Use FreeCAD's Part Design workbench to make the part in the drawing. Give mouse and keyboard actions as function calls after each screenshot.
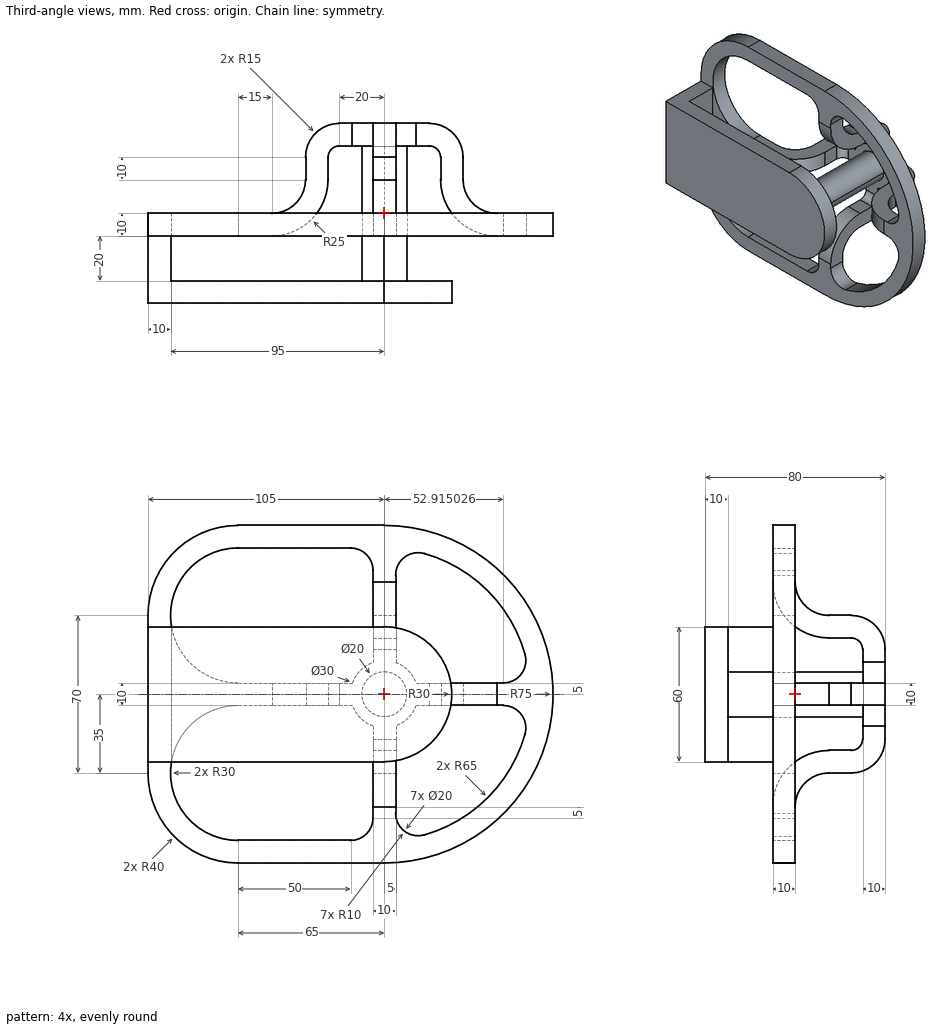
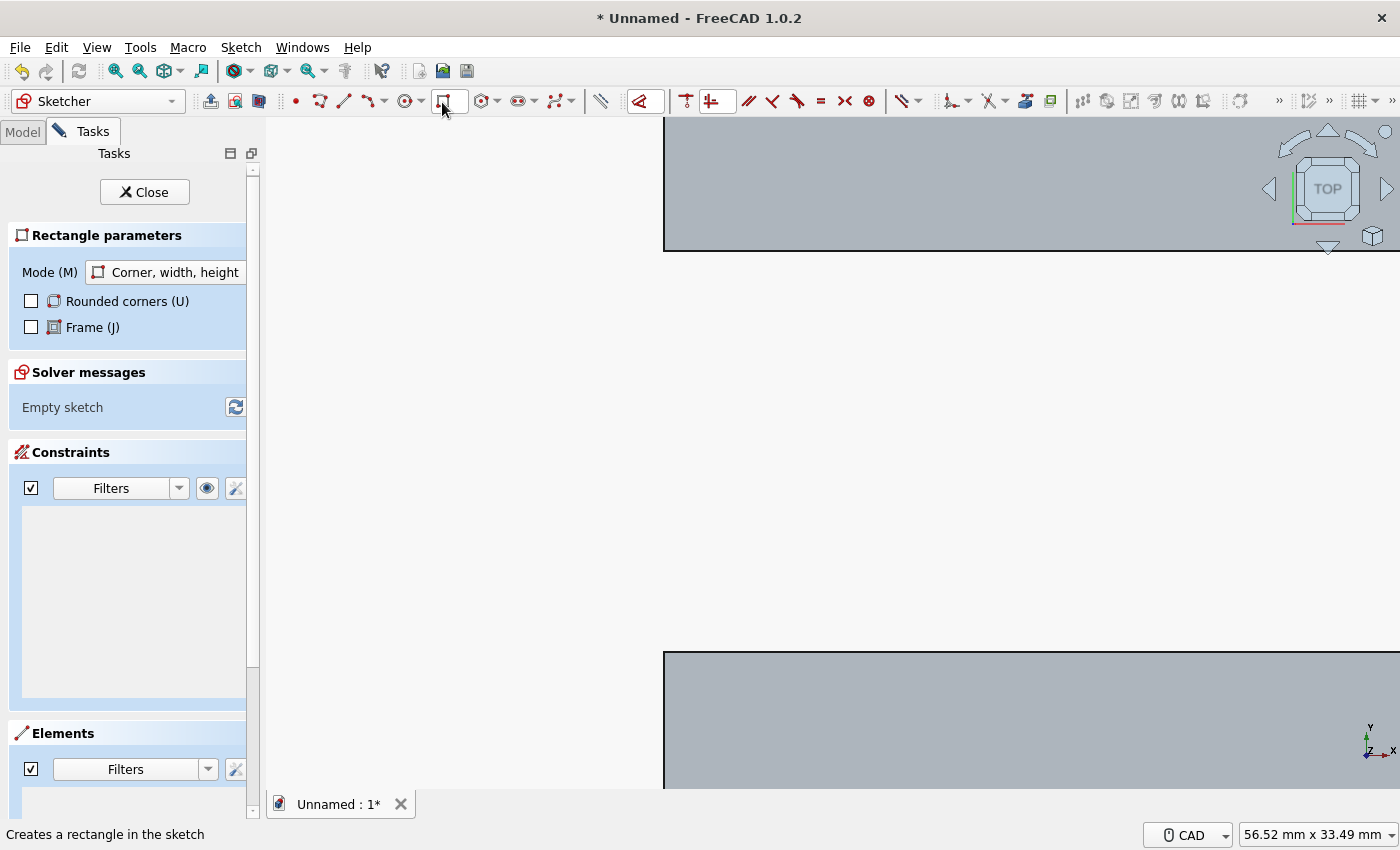
click(664, 251)
move(865, 652)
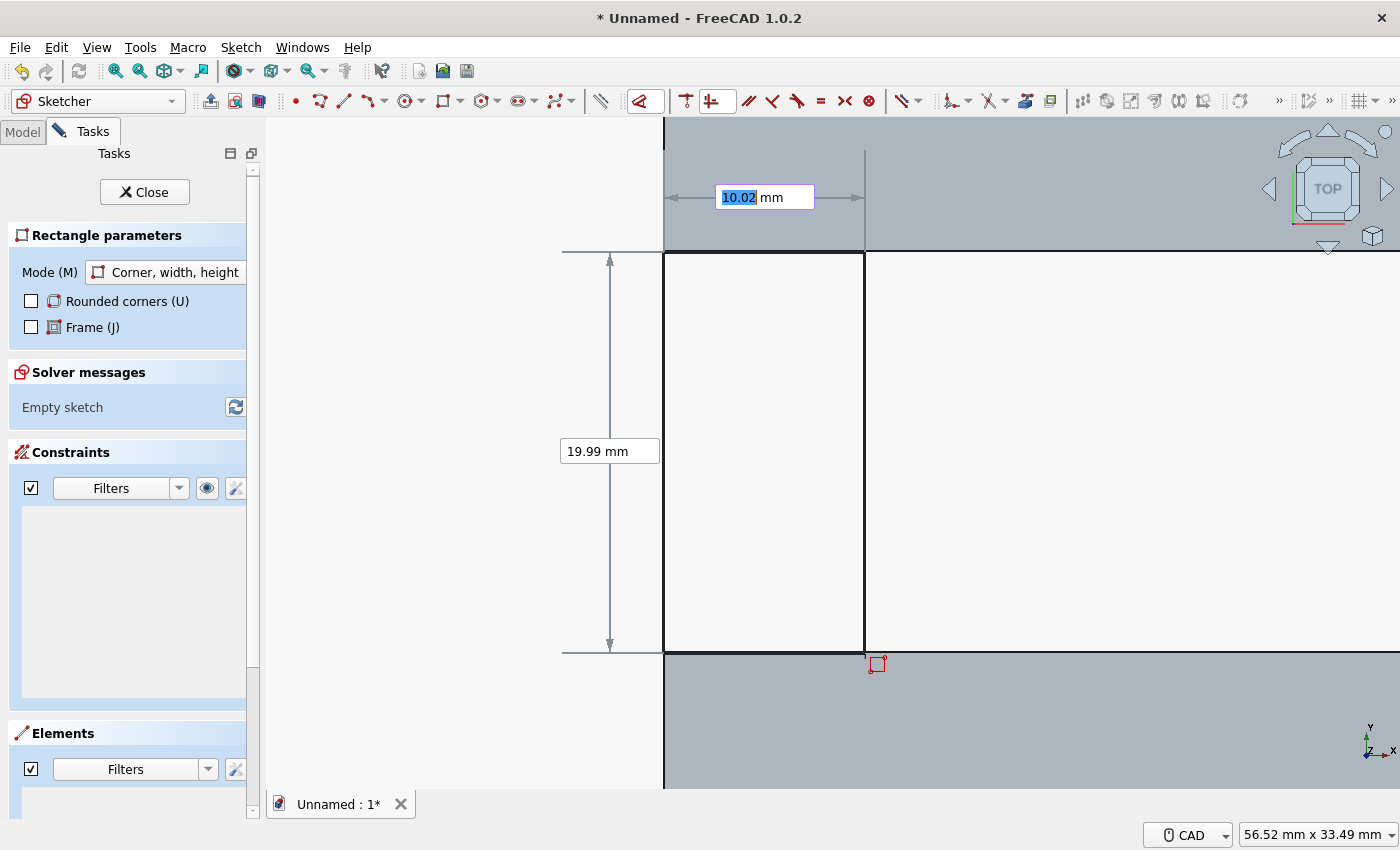
text(10)
key(Tab)
text(20)
key(Return)
key(Escape)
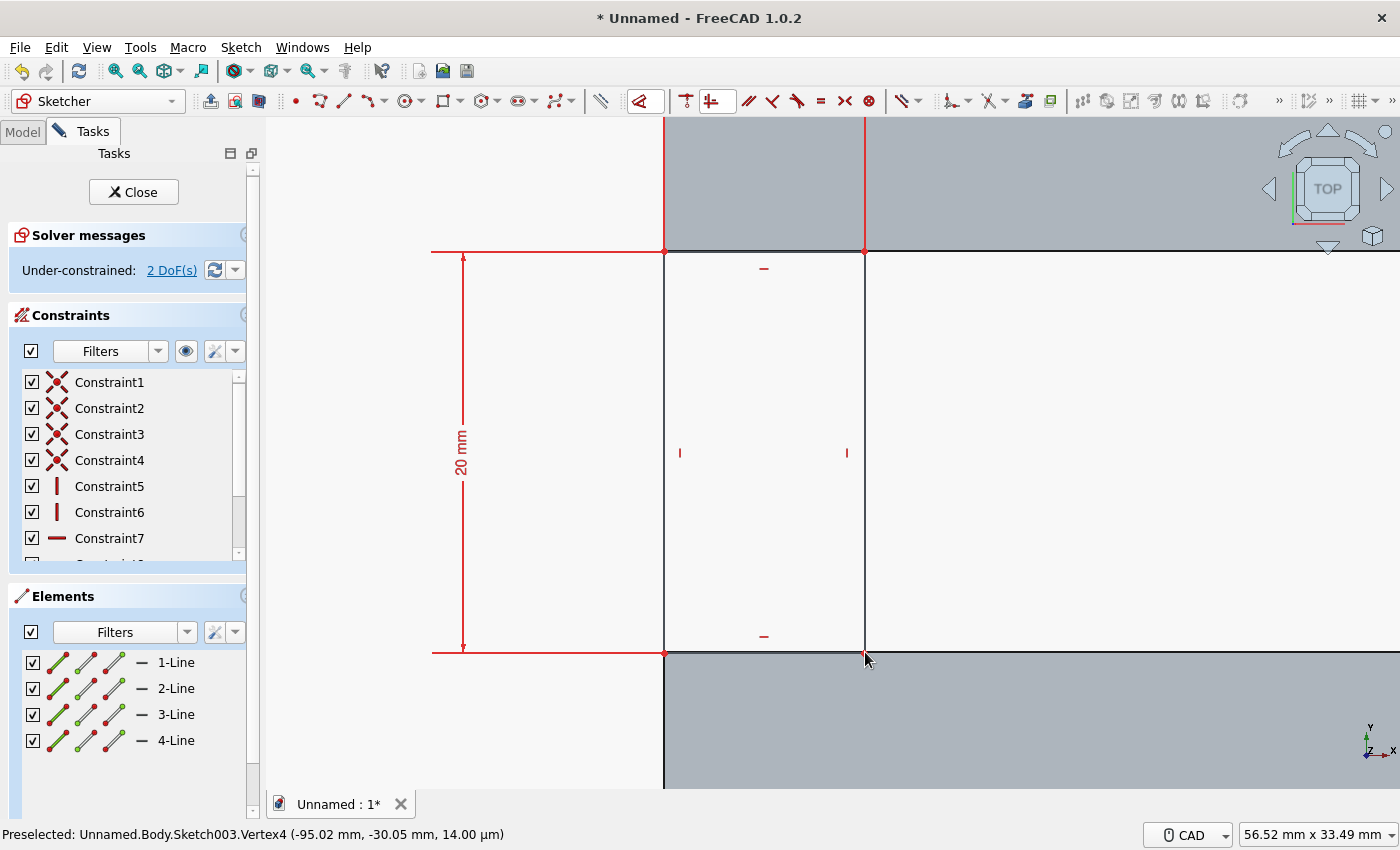
click(664, 252)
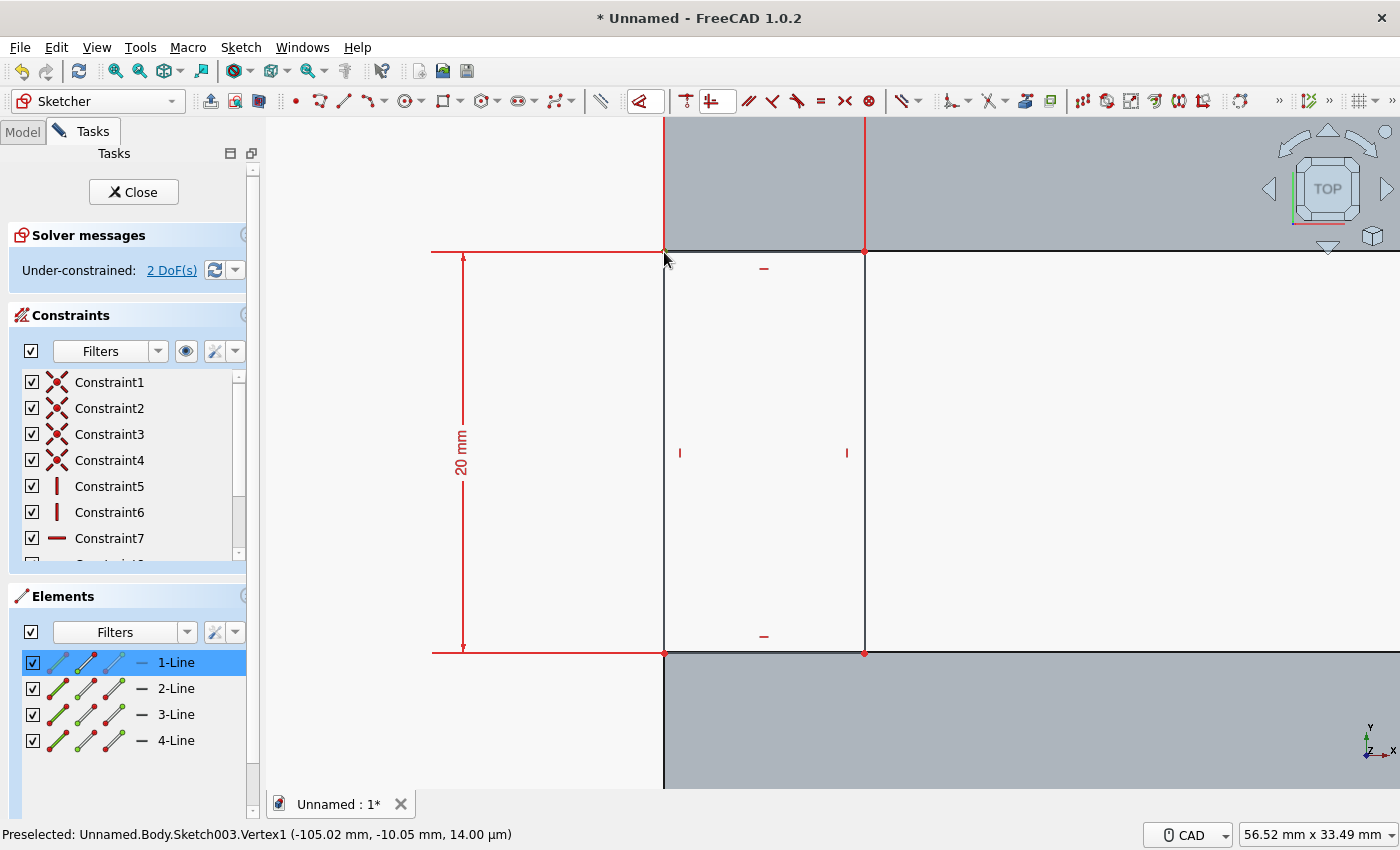
key(i)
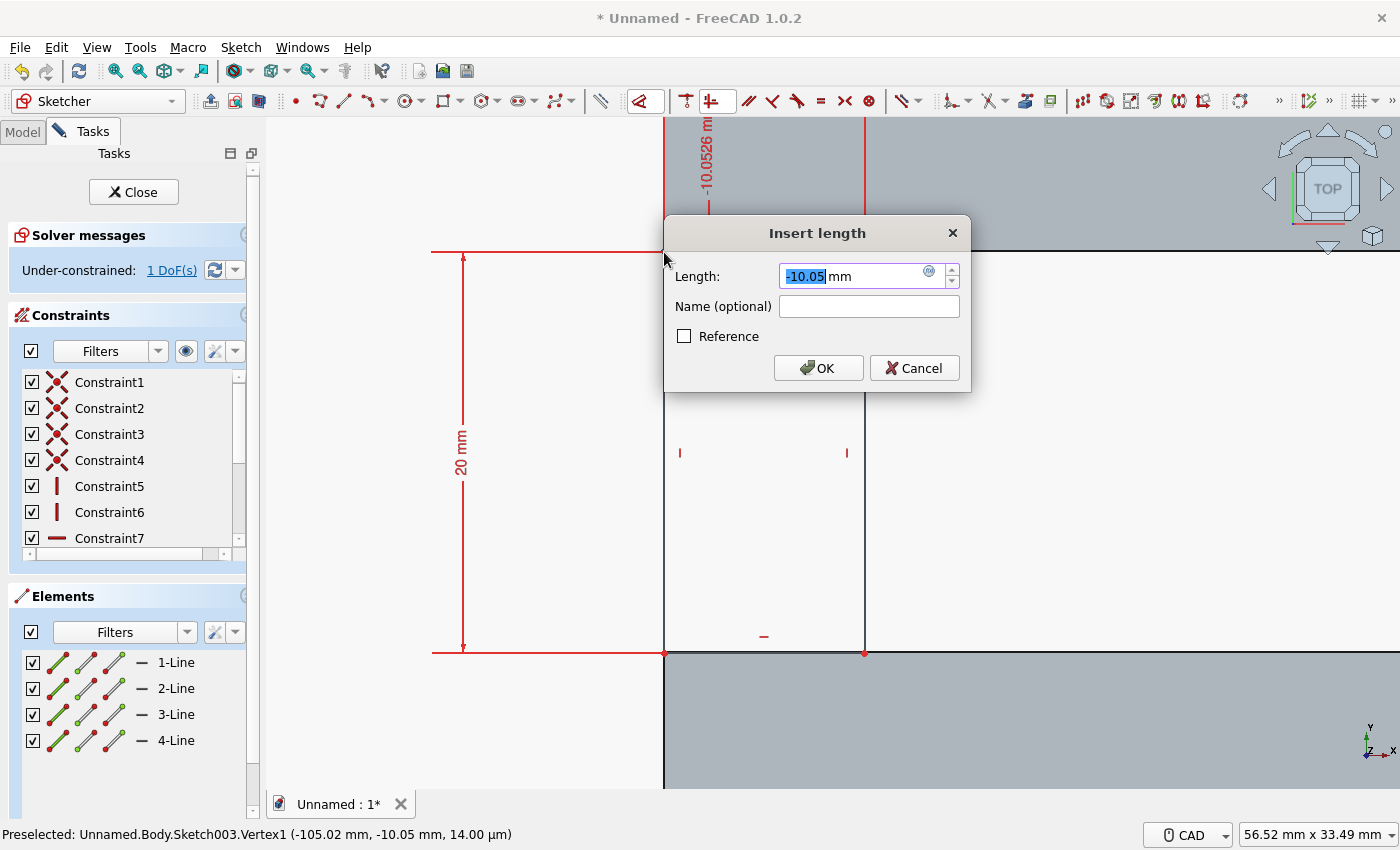
text(-10)
key(Return)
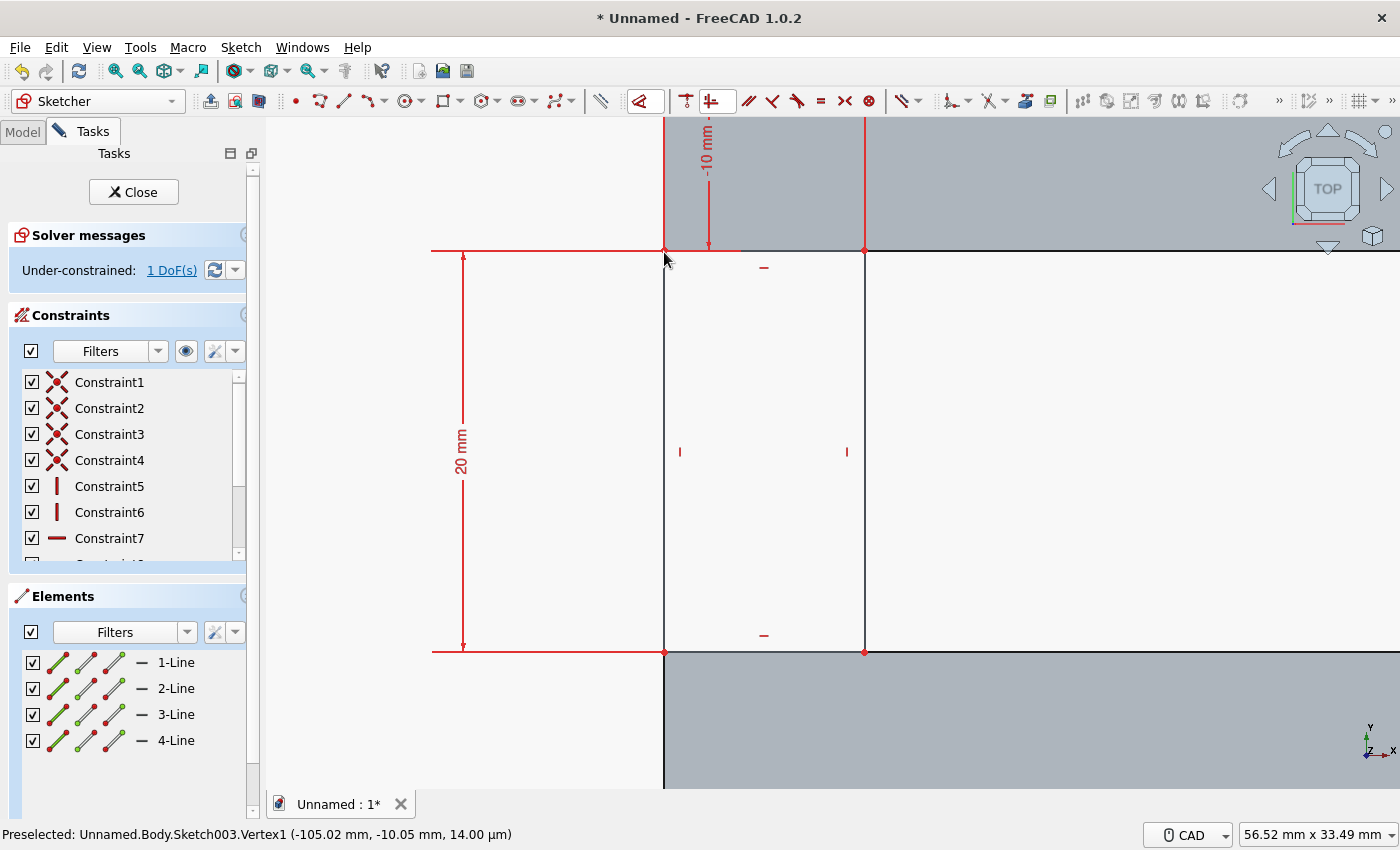
click(865, 652)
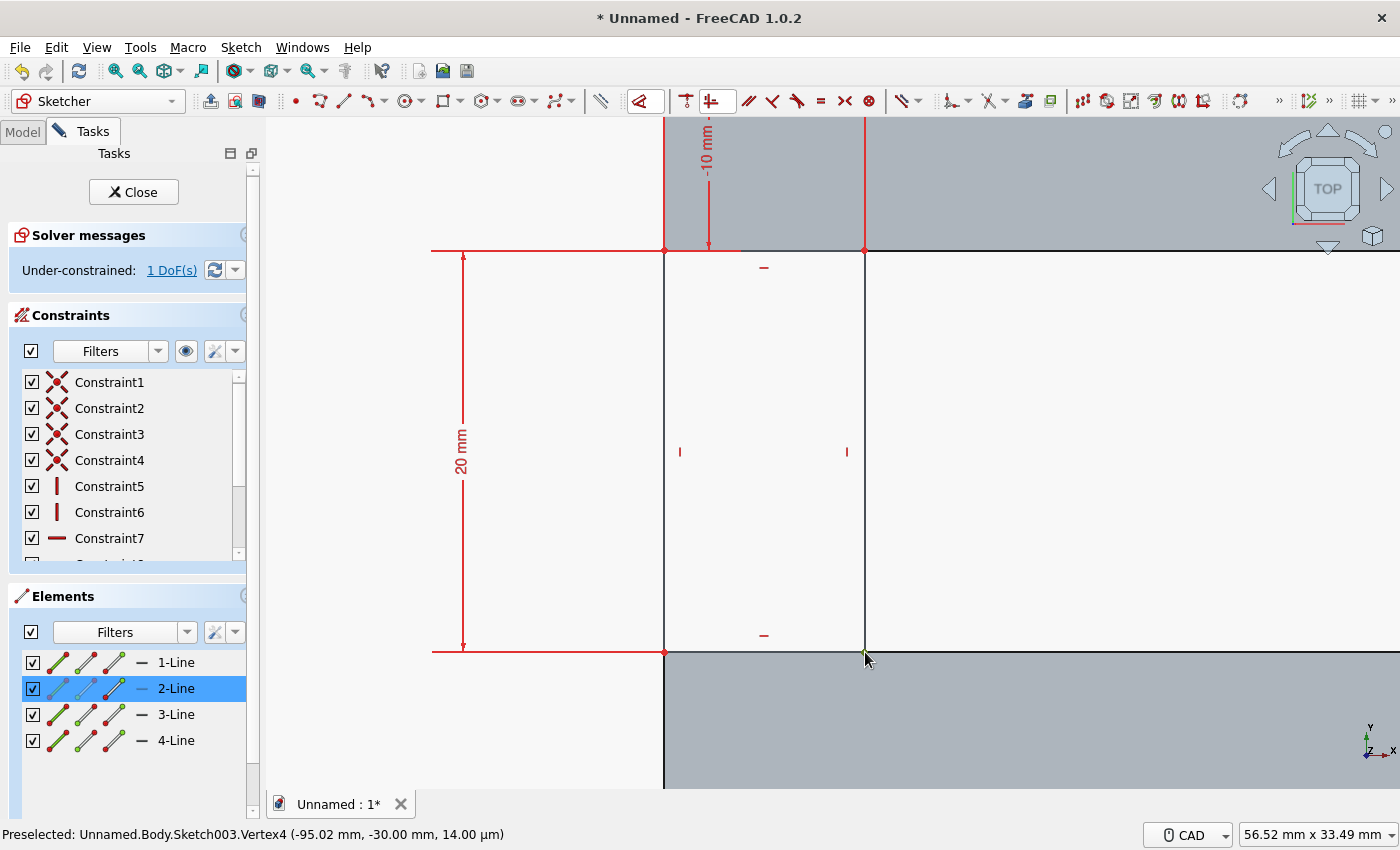
click(658, 102)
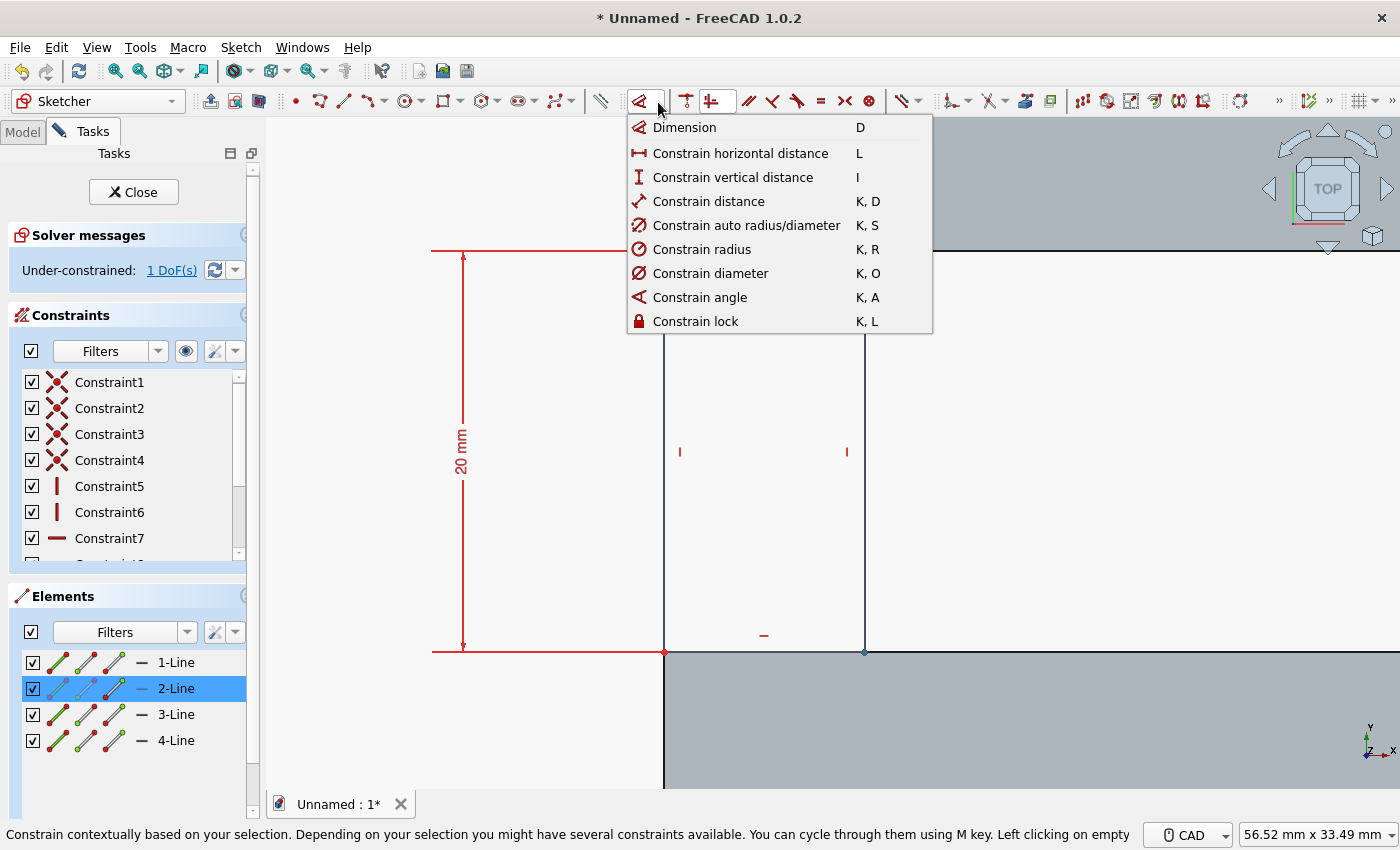
click(780, 153)